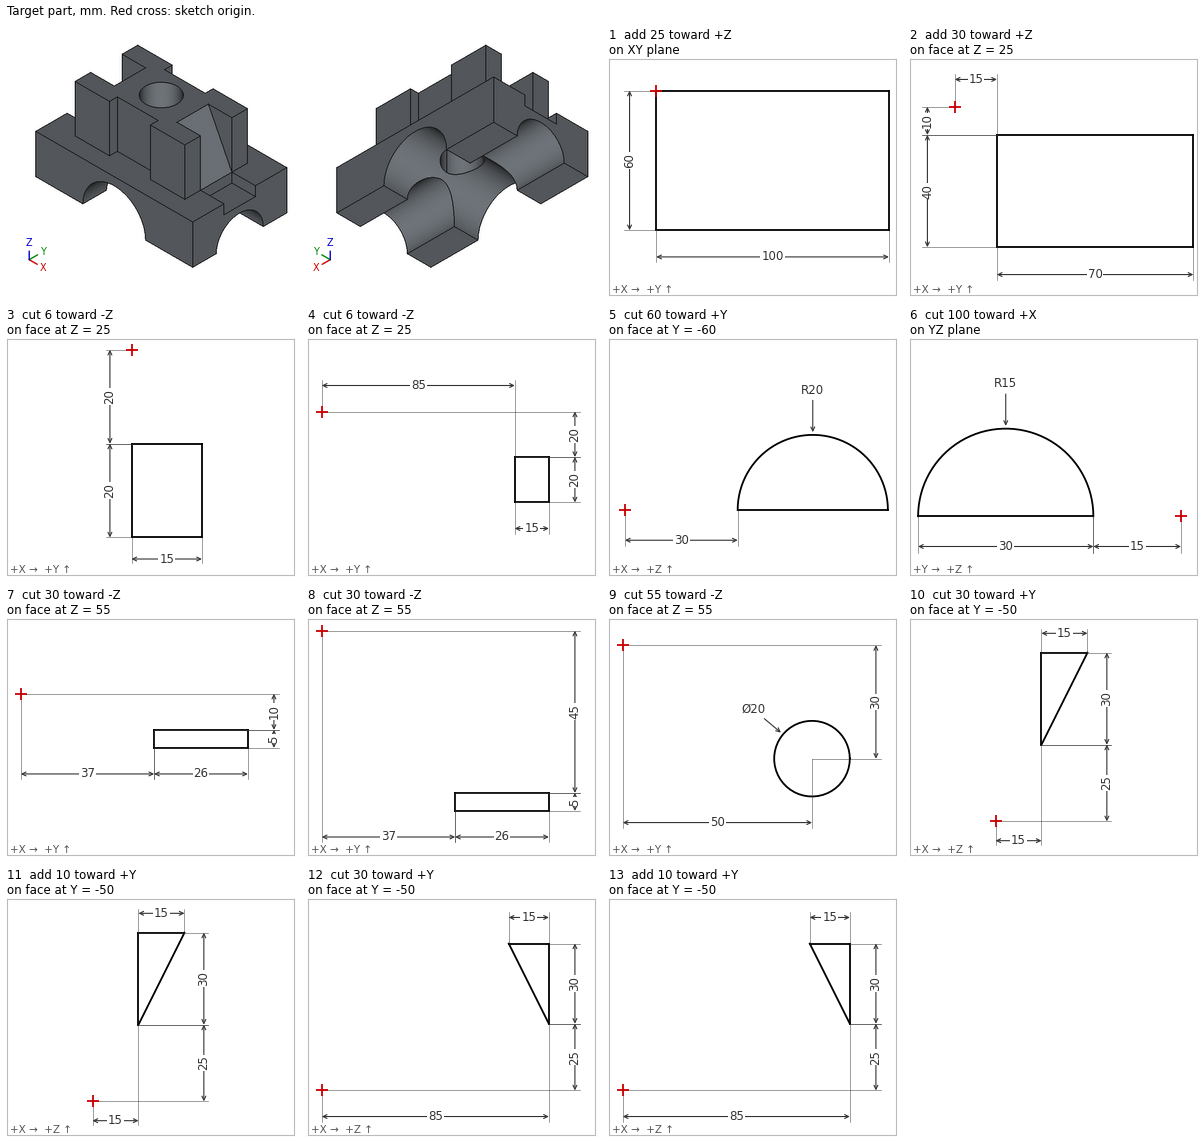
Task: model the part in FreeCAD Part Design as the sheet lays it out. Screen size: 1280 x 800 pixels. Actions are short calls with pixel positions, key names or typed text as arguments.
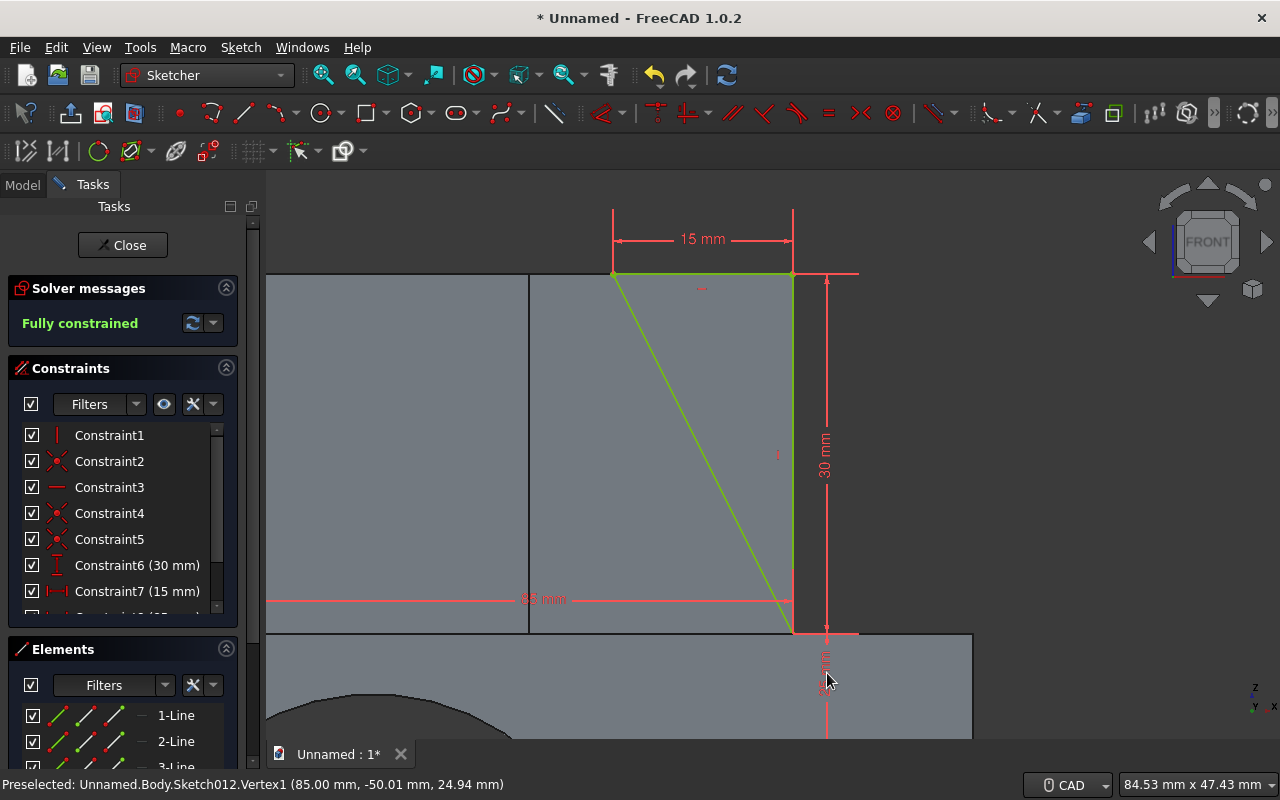
click(123, 245)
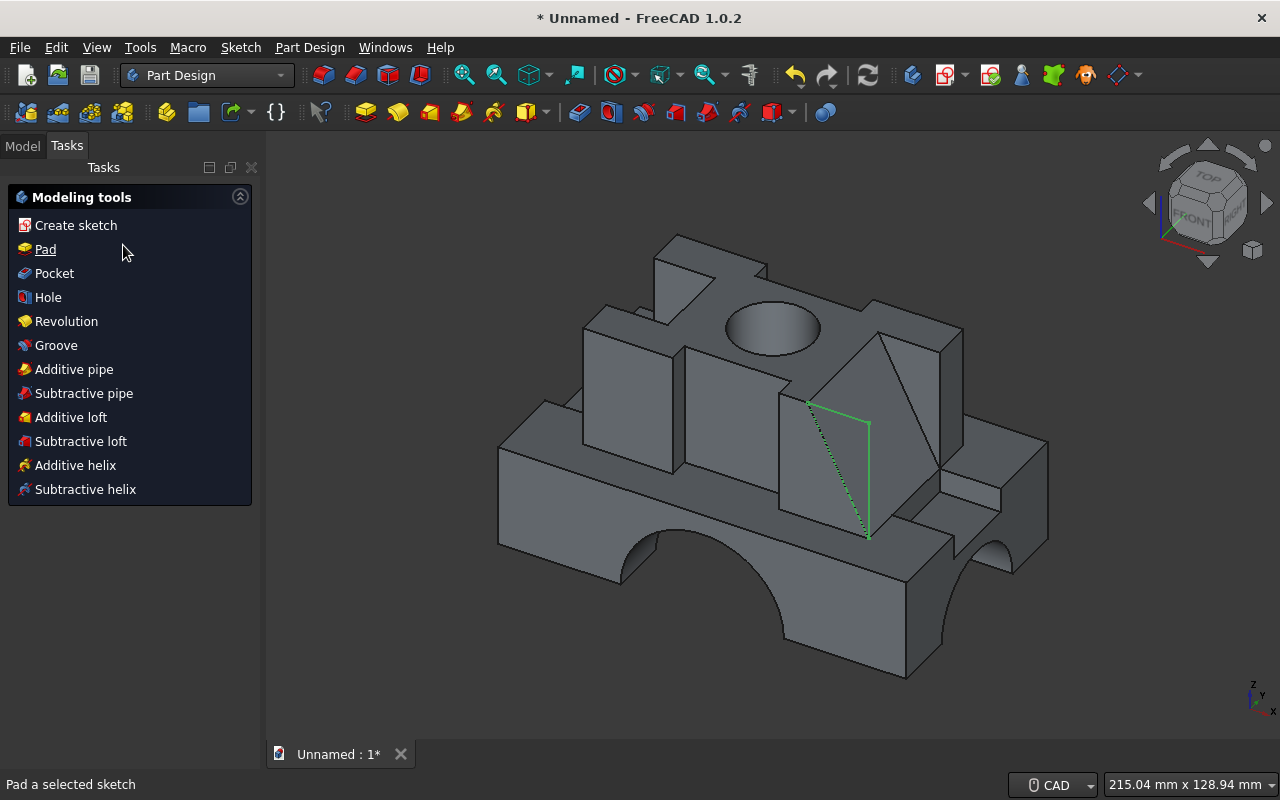
click(366, 112)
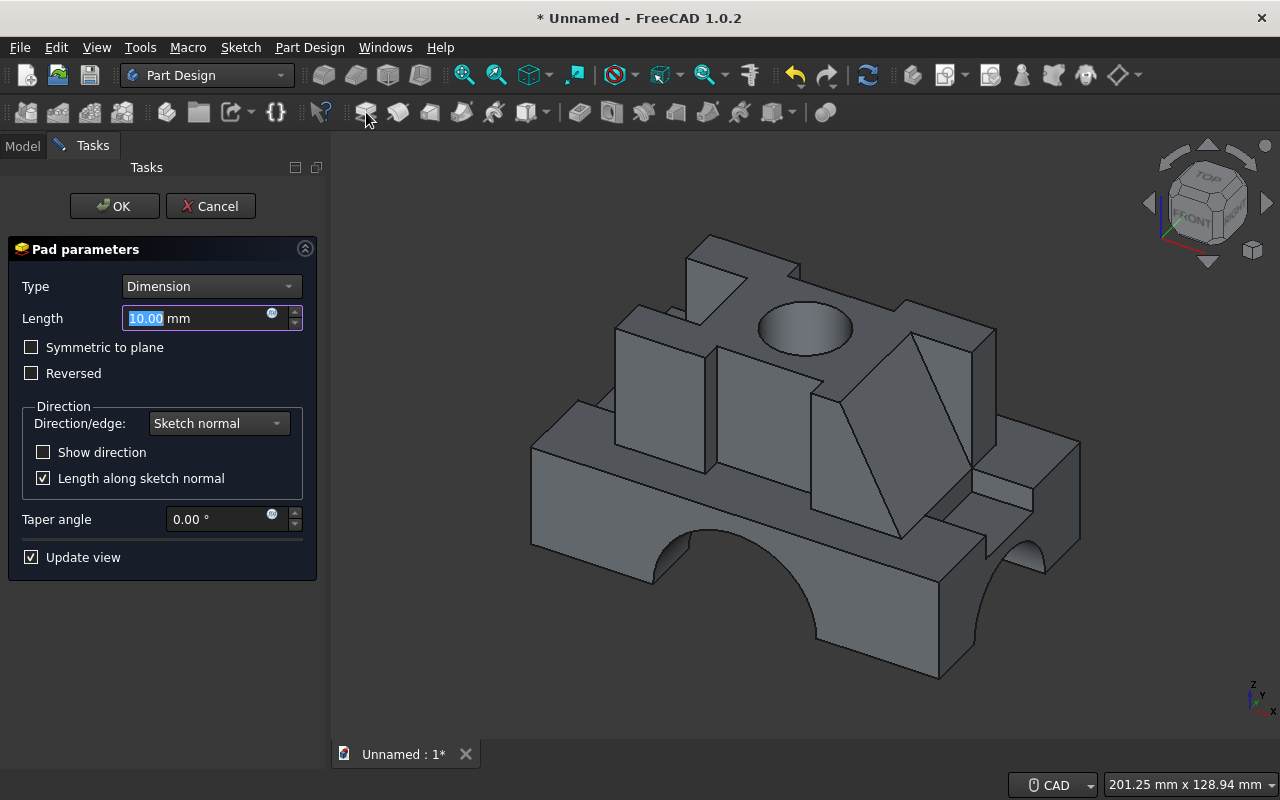
text(10)
key(Tab)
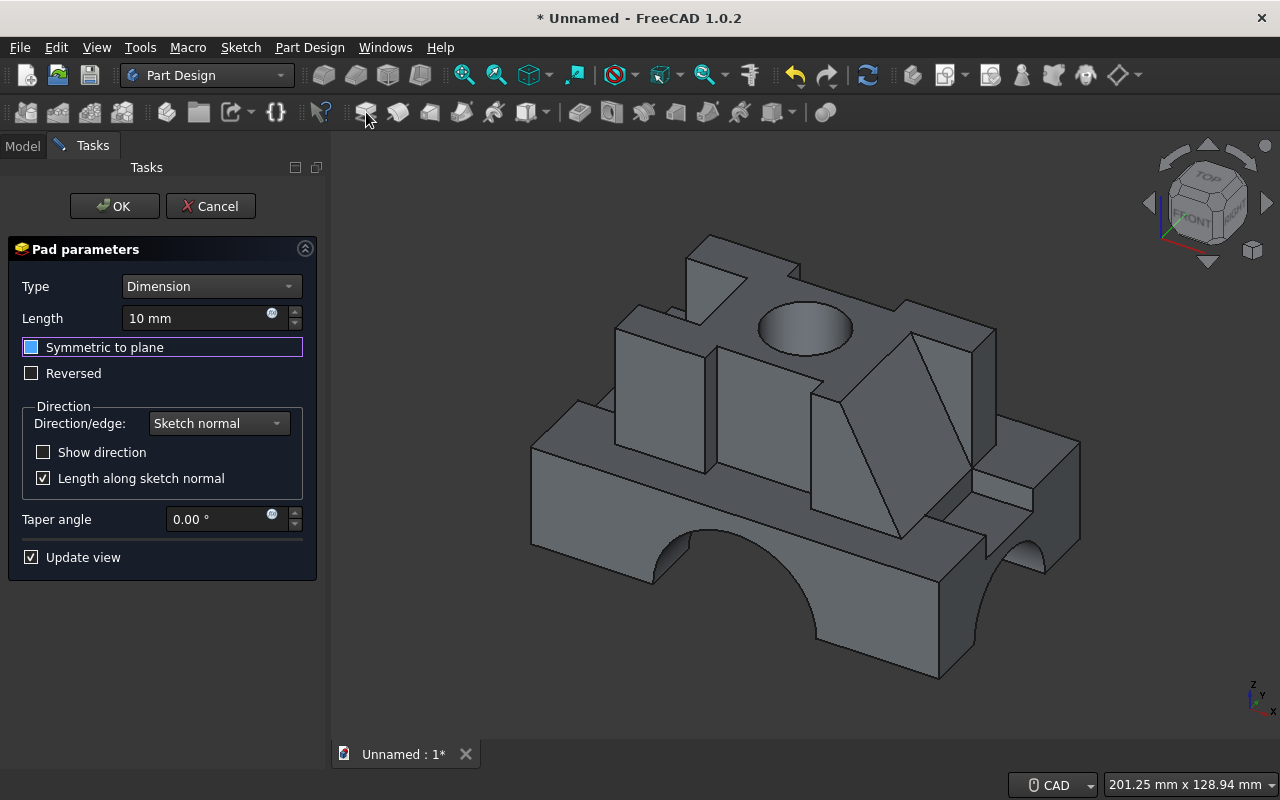
click(30, 373)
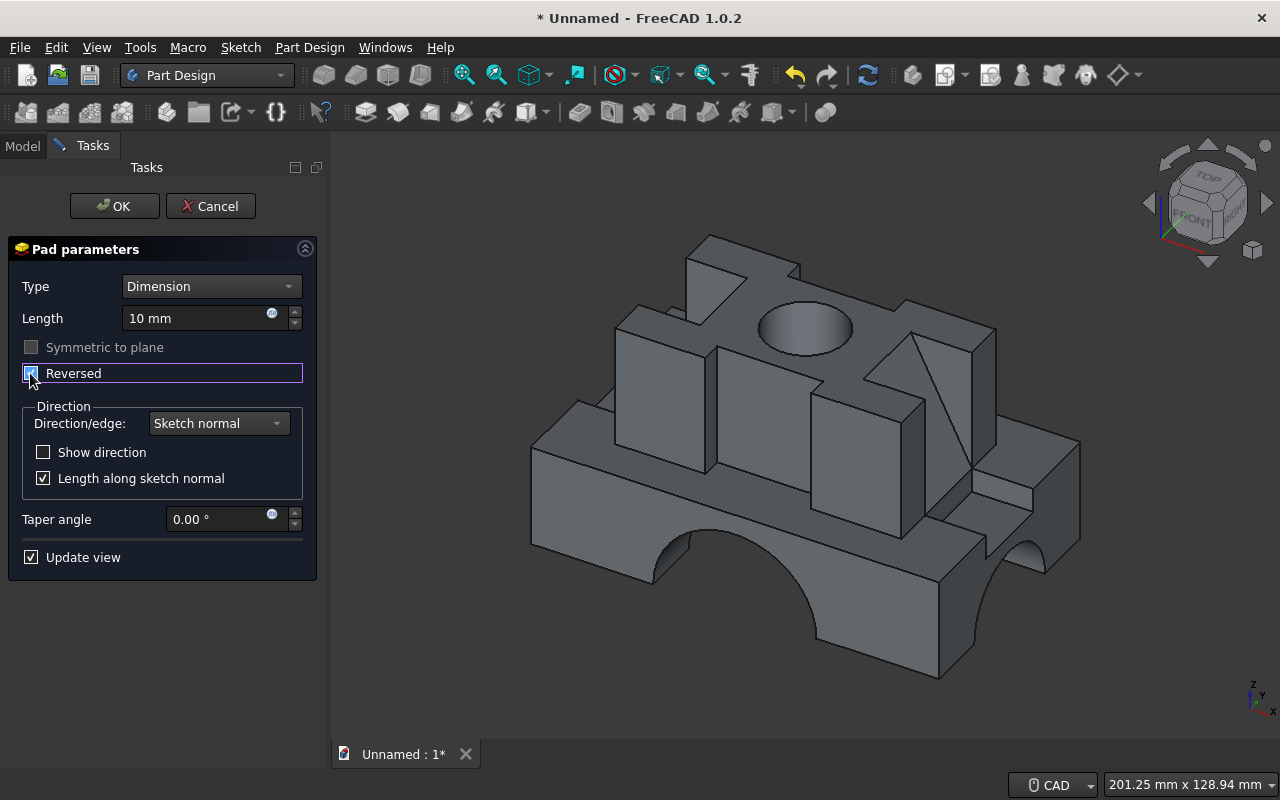
click(115, 206)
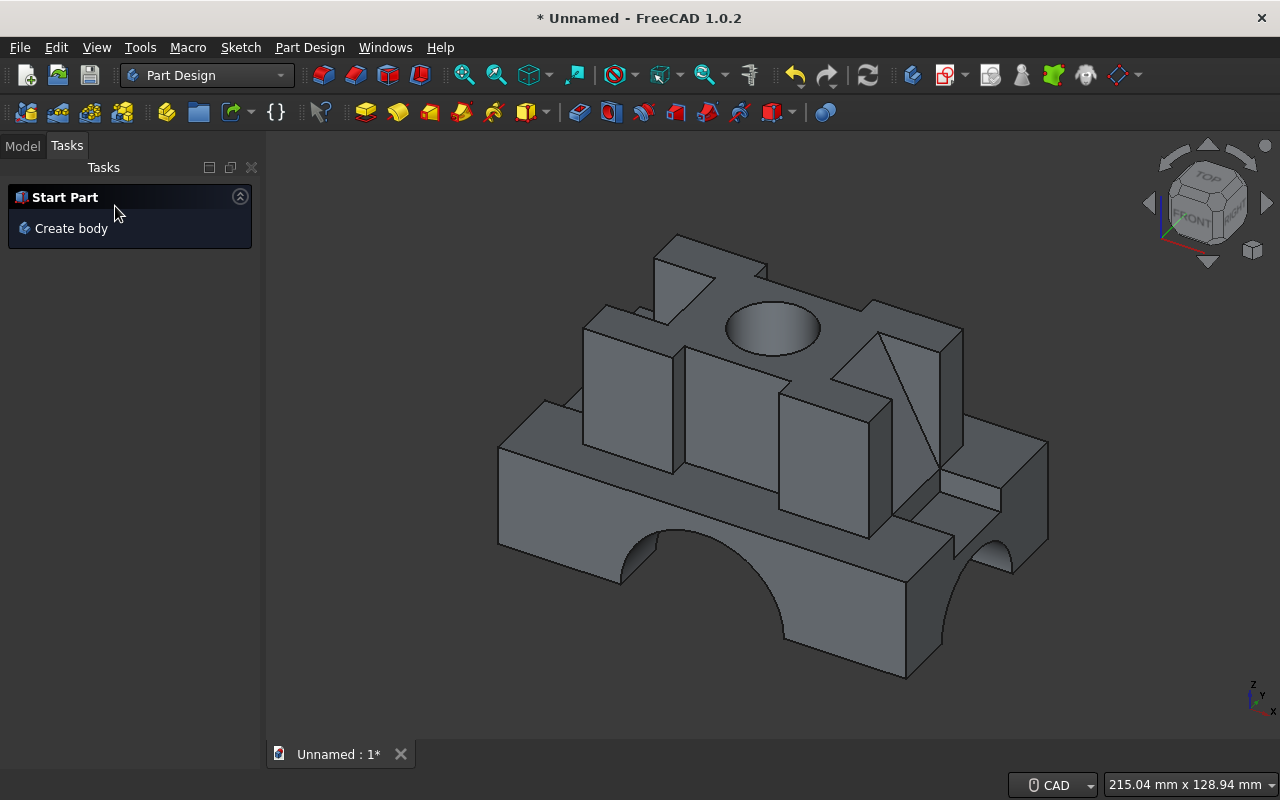
key(0)